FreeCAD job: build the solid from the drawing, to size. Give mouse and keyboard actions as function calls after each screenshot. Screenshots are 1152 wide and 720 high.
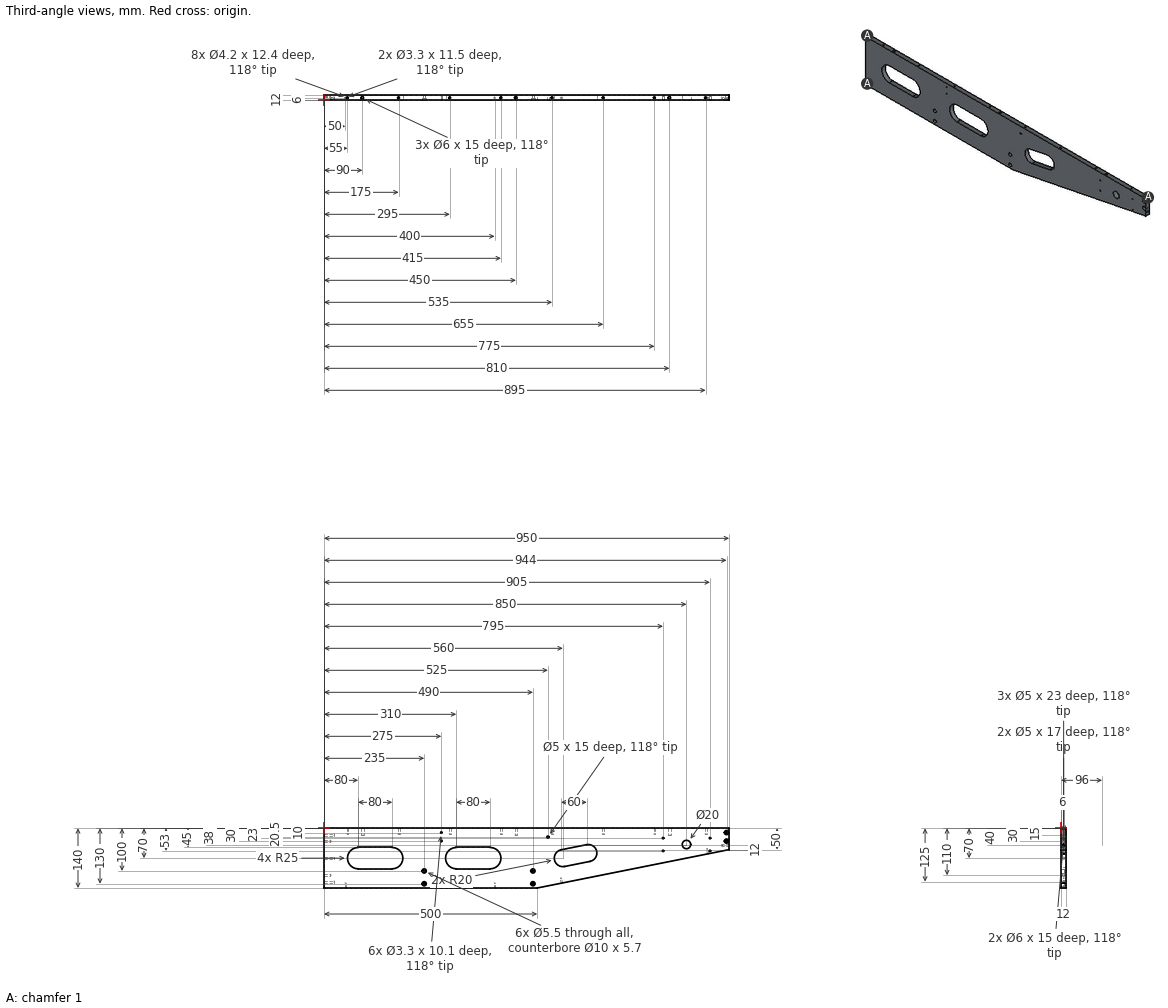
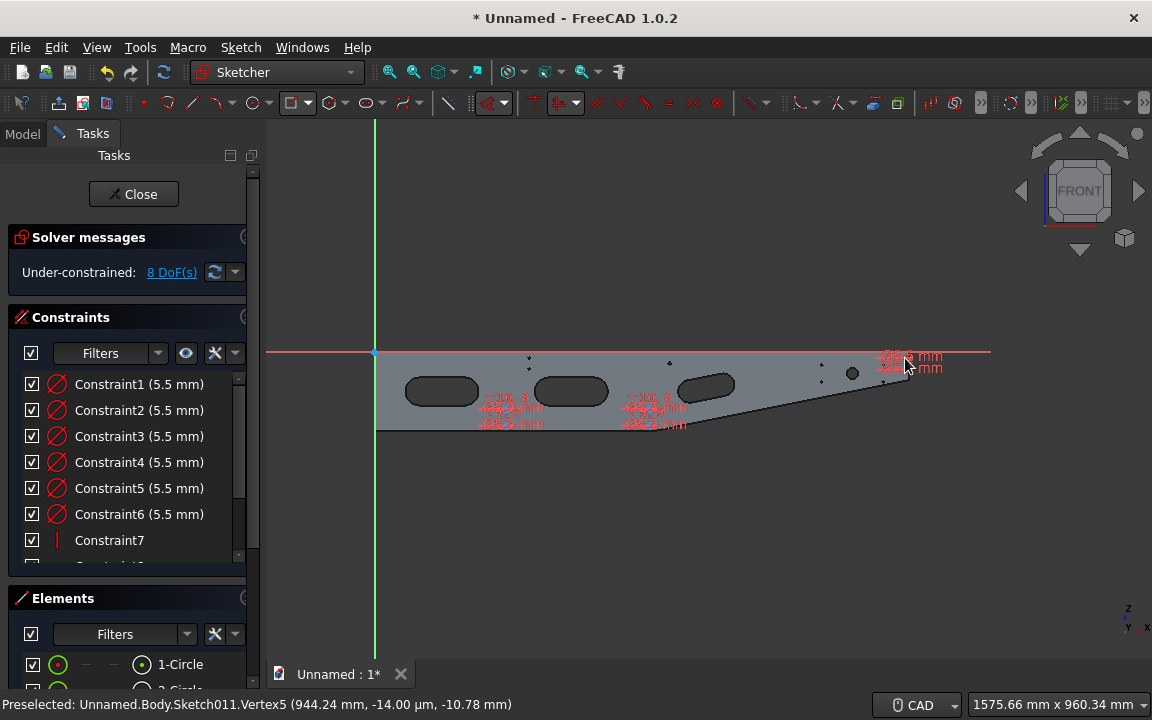
click(905, 370)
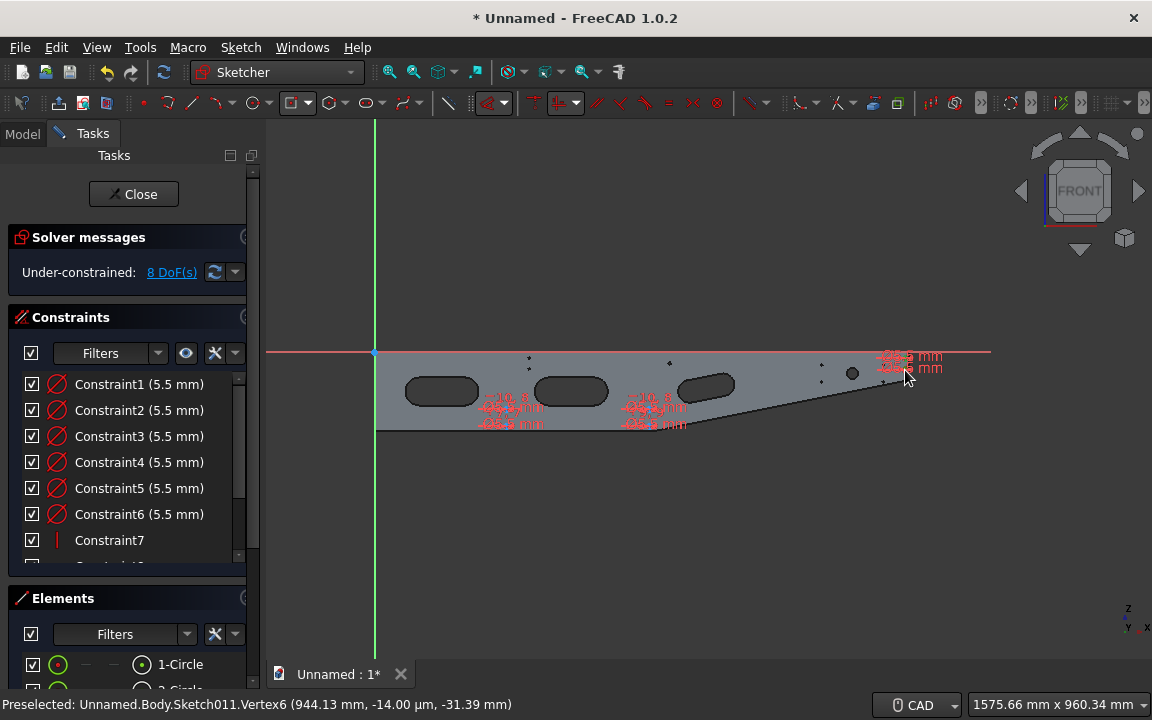
key(v)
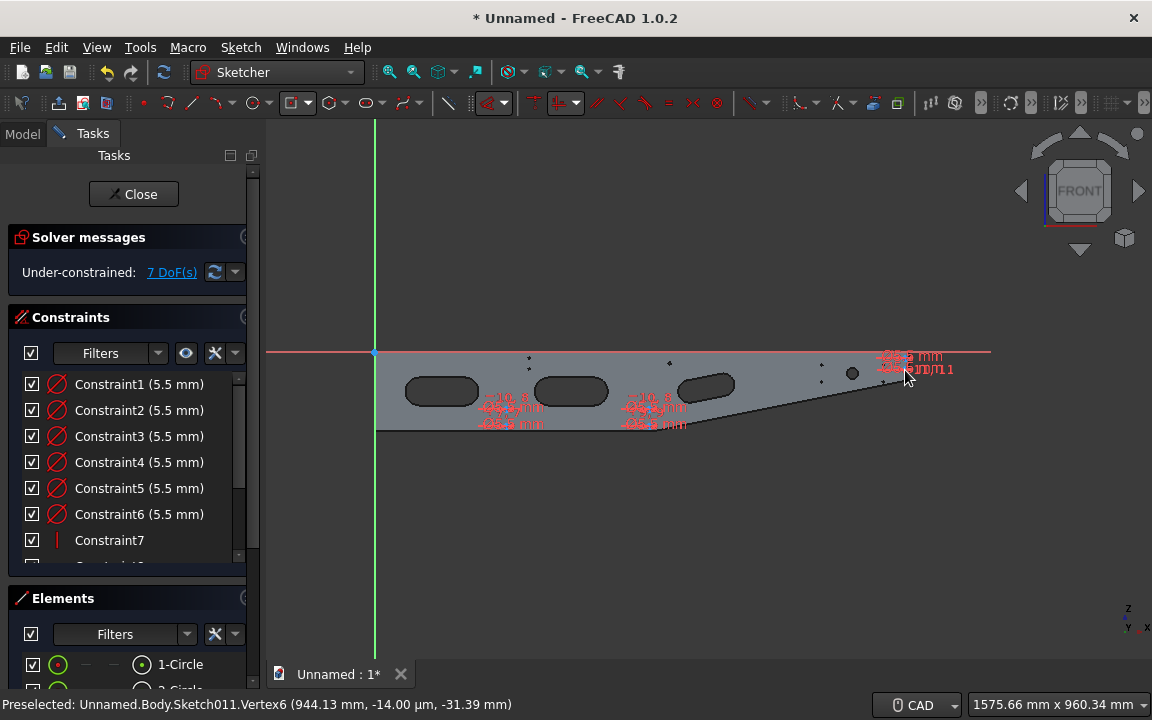
scroll(905, 358, up, 10)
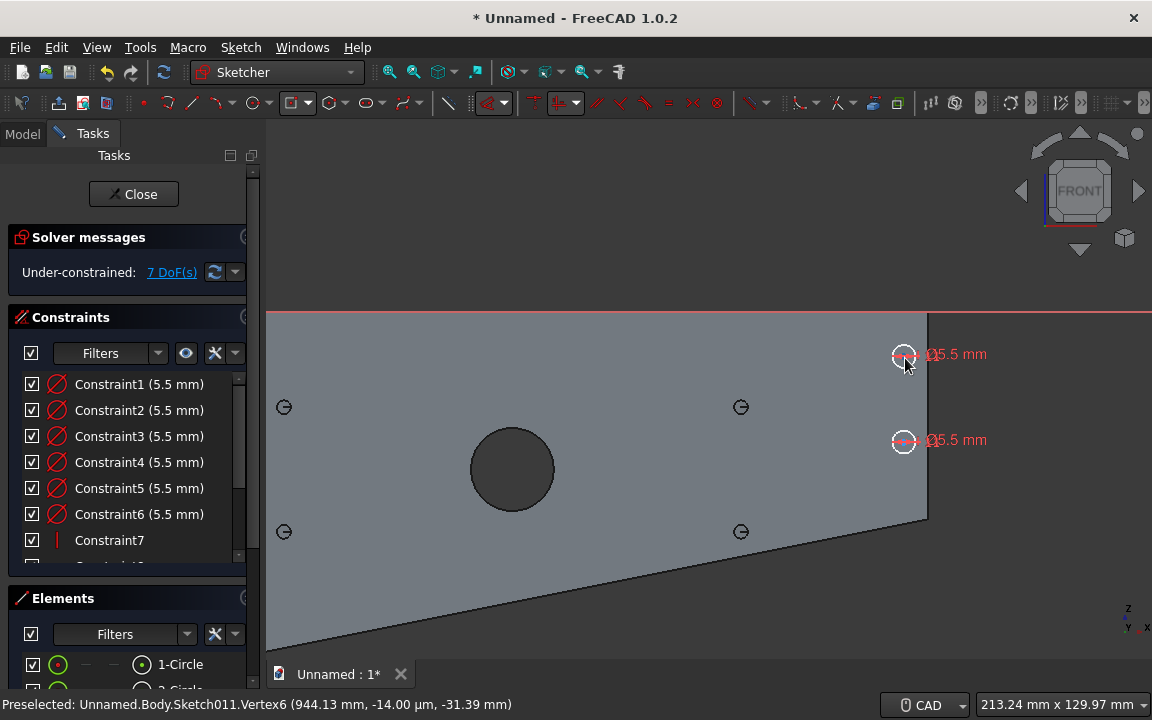
click(904, 356)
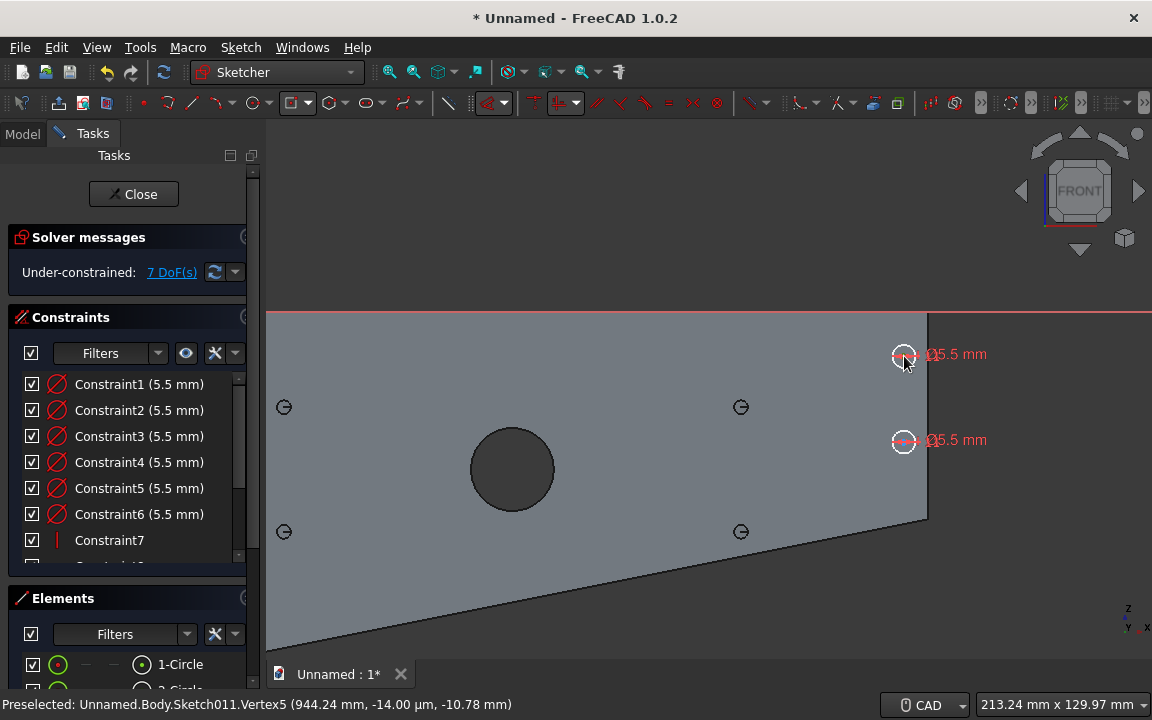
key(i)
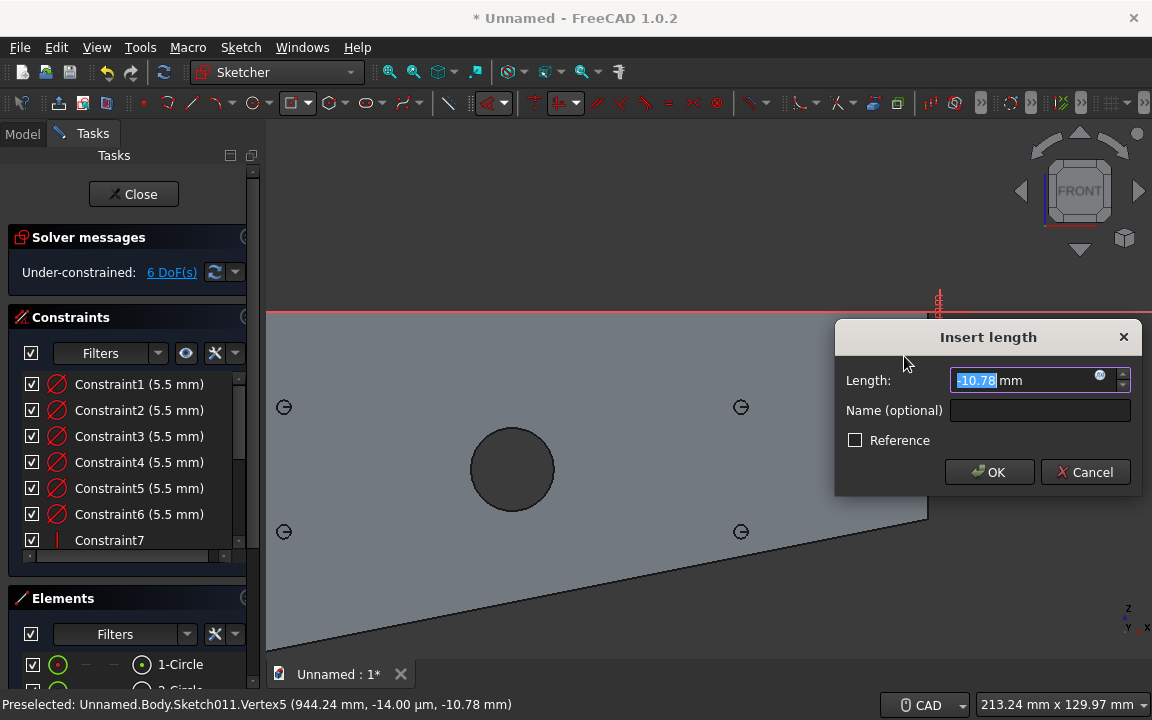
text(-10)
key(Return)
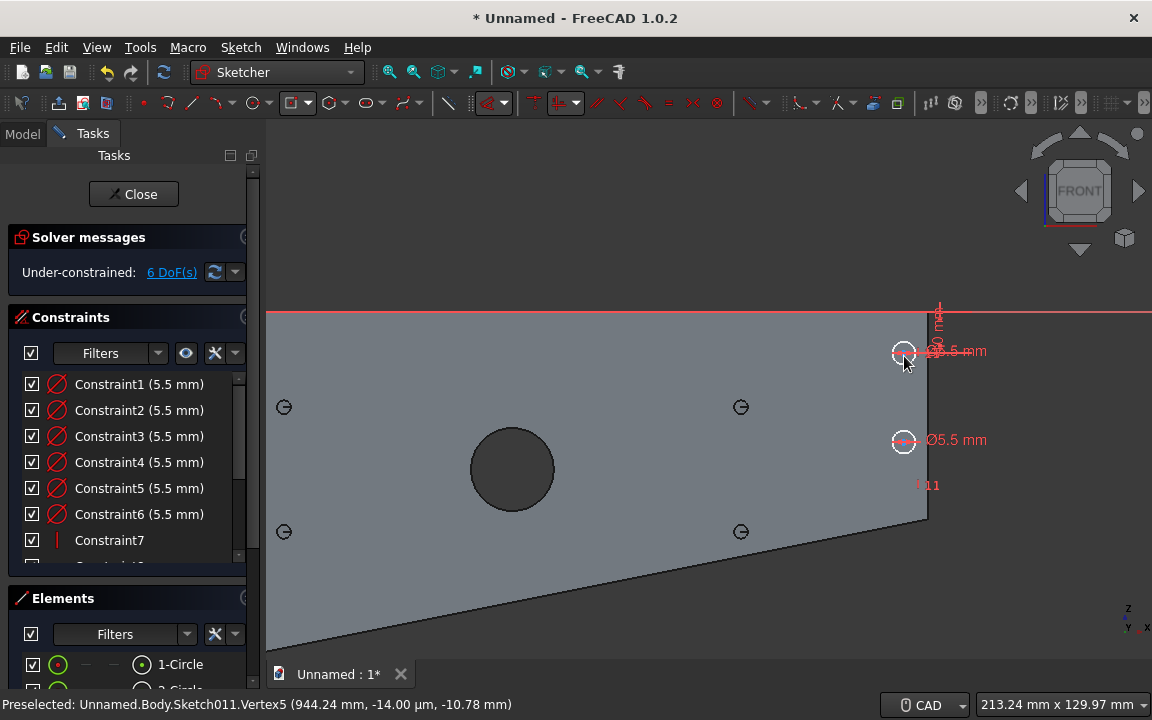
scroll(905, 358, down, 10)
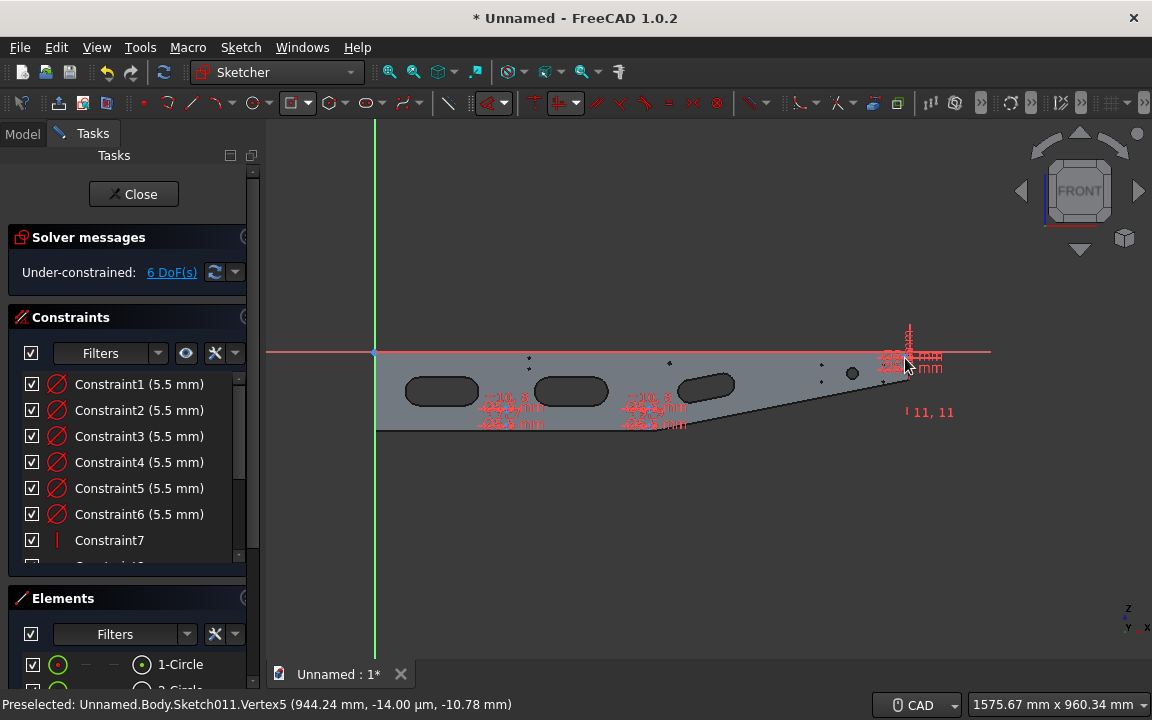
scroll(905, 370, up, 5)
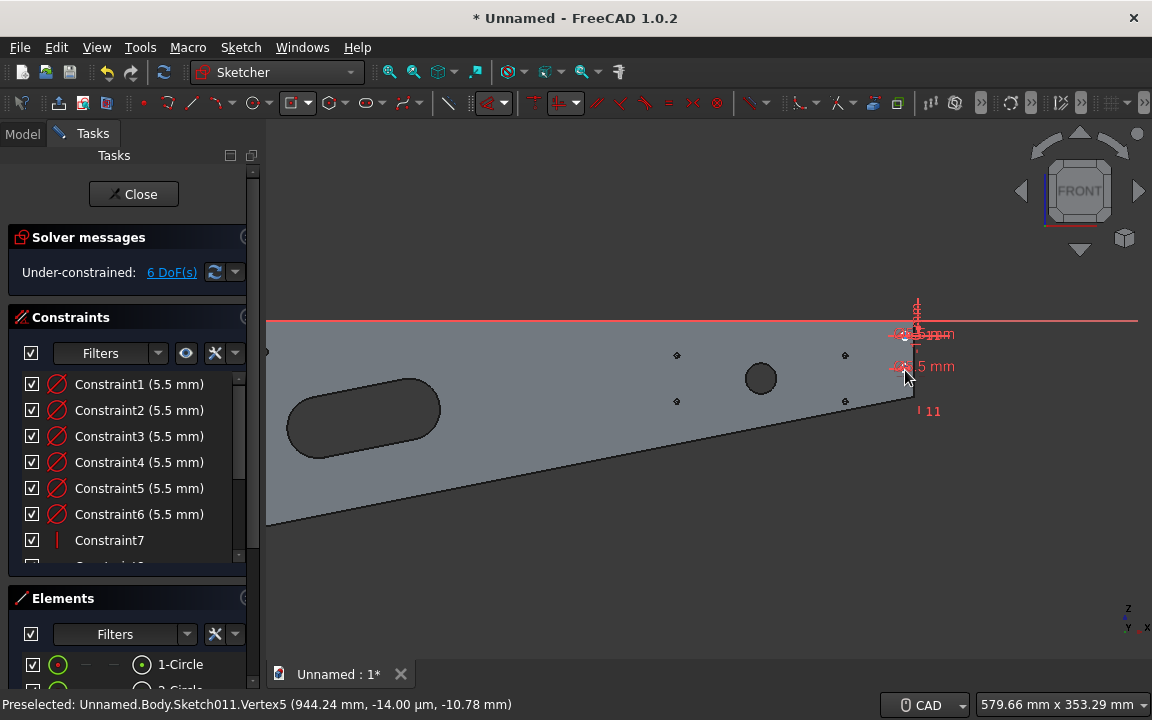
click(905, 369)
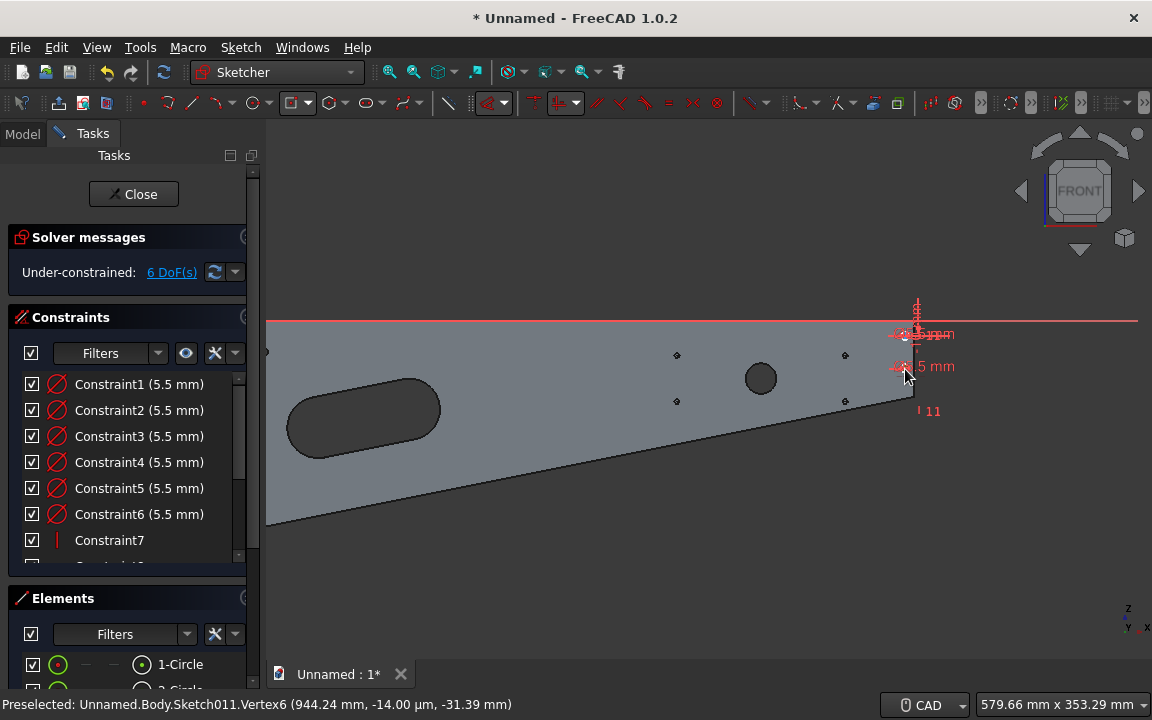
key(i)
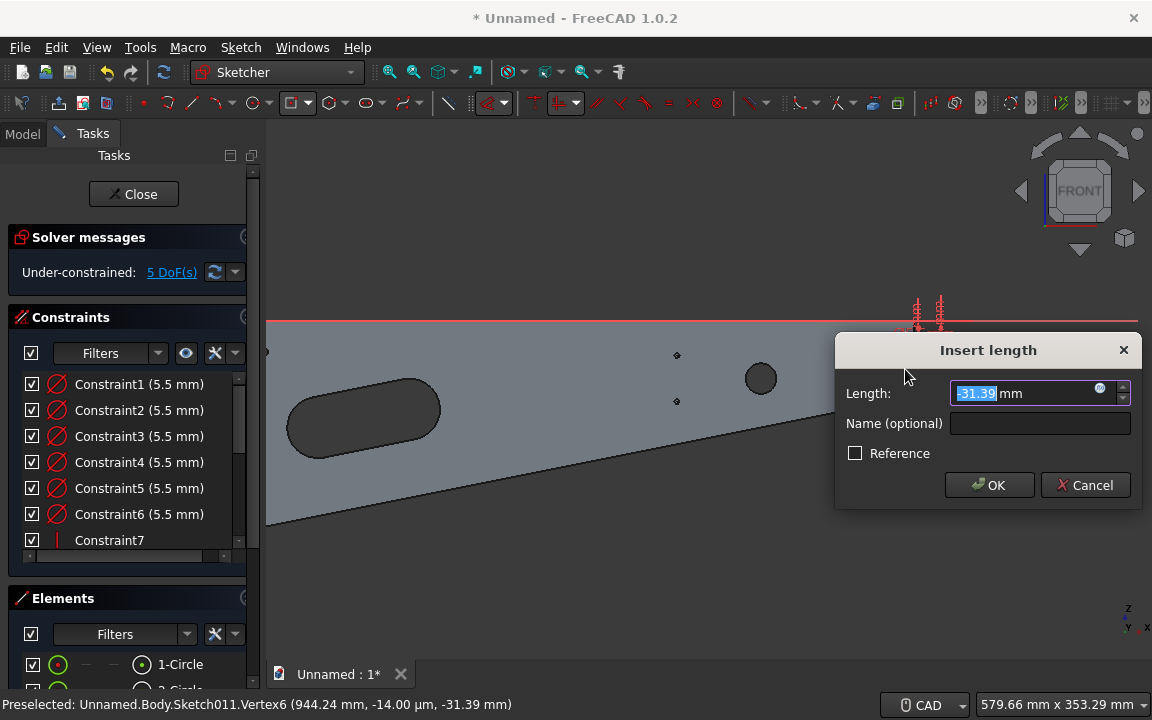
text(-30)
key(Return)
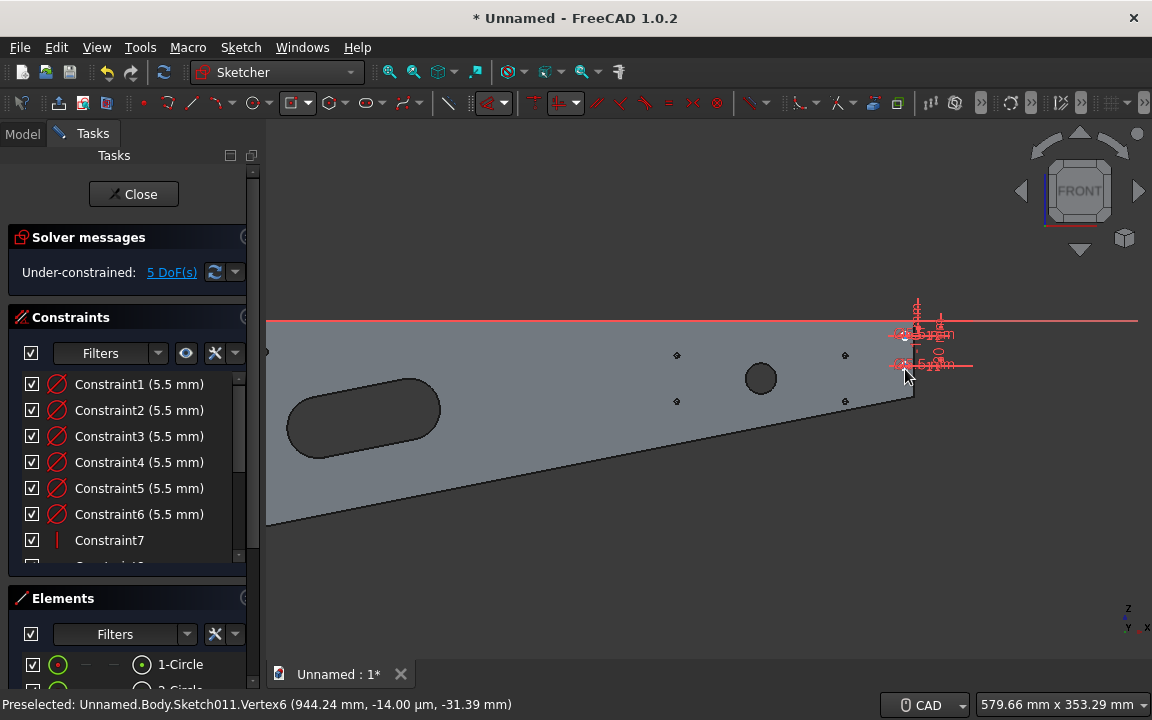
scroll(905, 370, down, 5)